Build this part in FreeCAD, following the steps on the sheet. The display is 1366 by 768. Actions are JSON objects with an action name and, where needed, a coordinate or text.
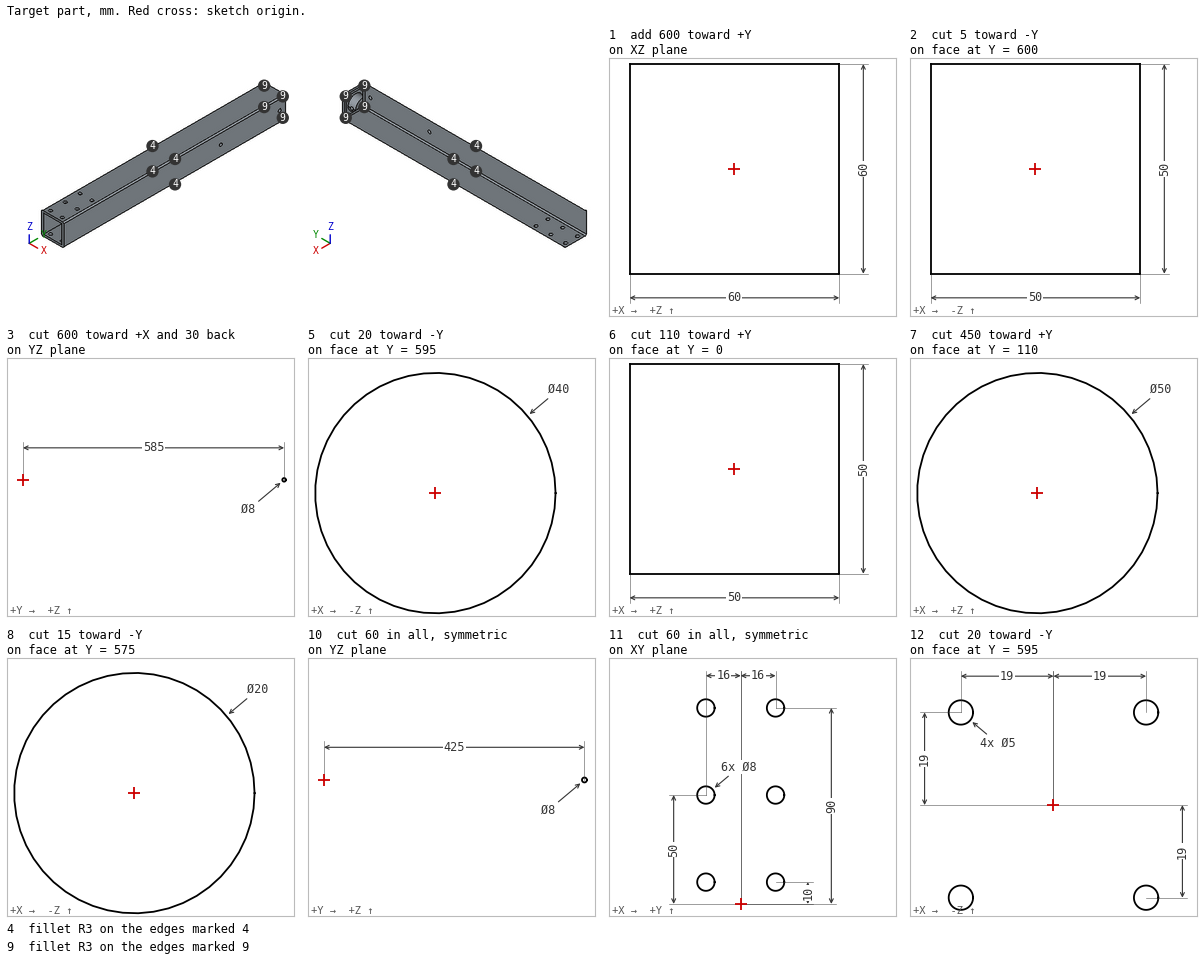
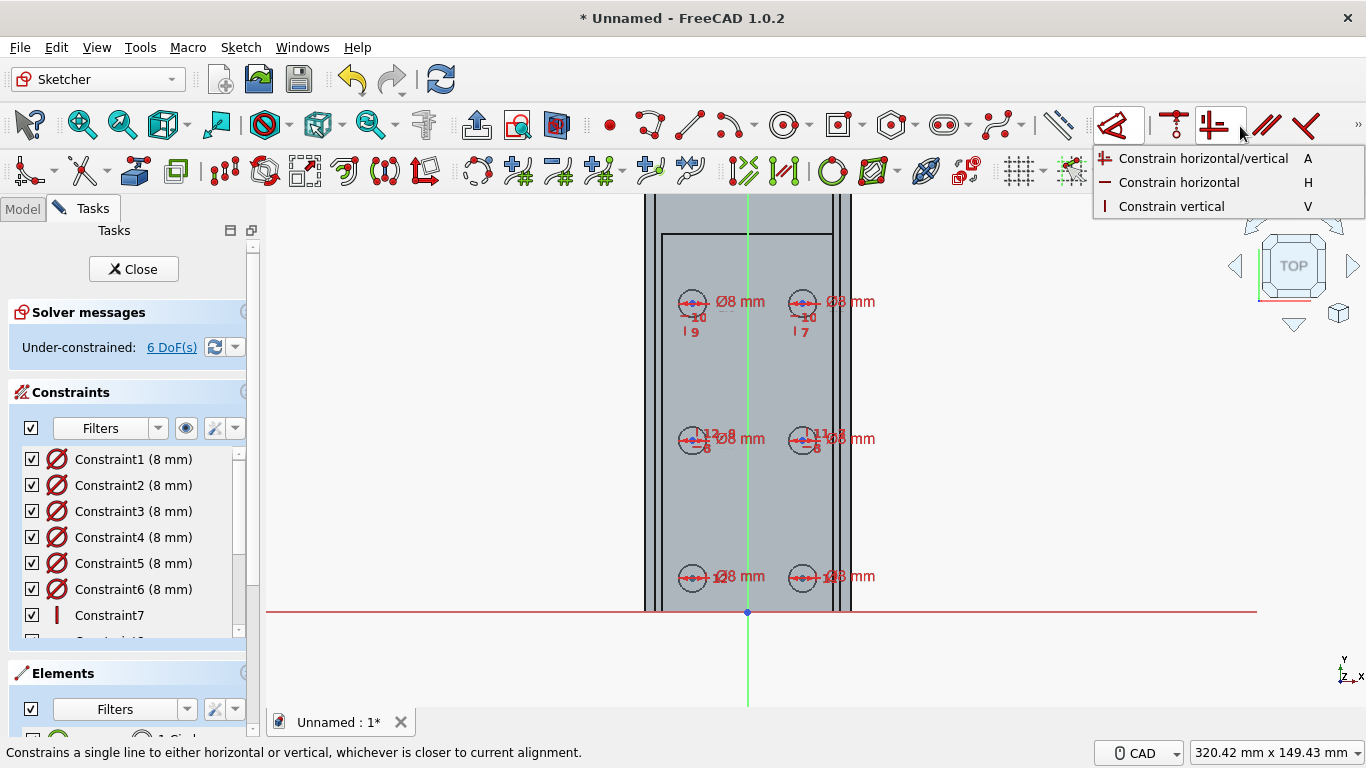
{"action": "left_click", "coordinate": [1229, 182]}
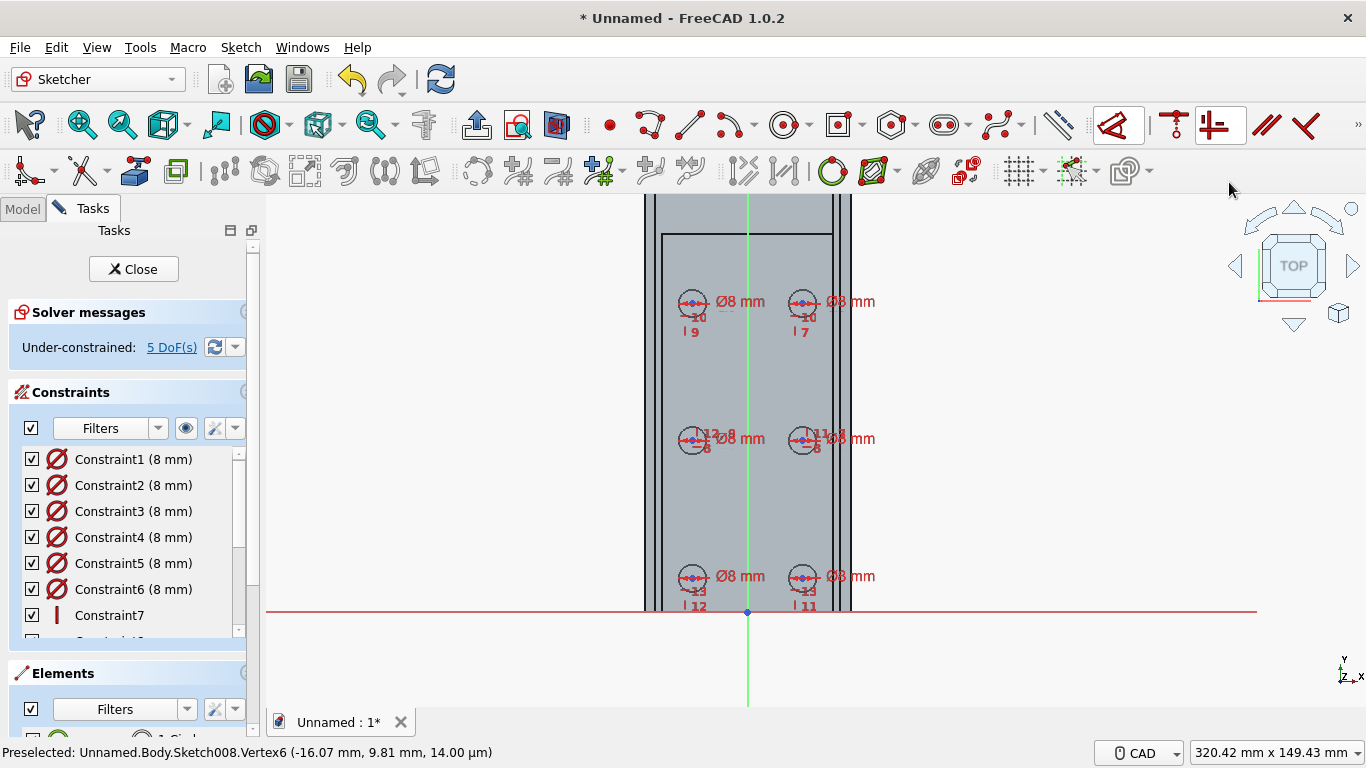
{"action": "left_click", "coordinate": [692, 441]}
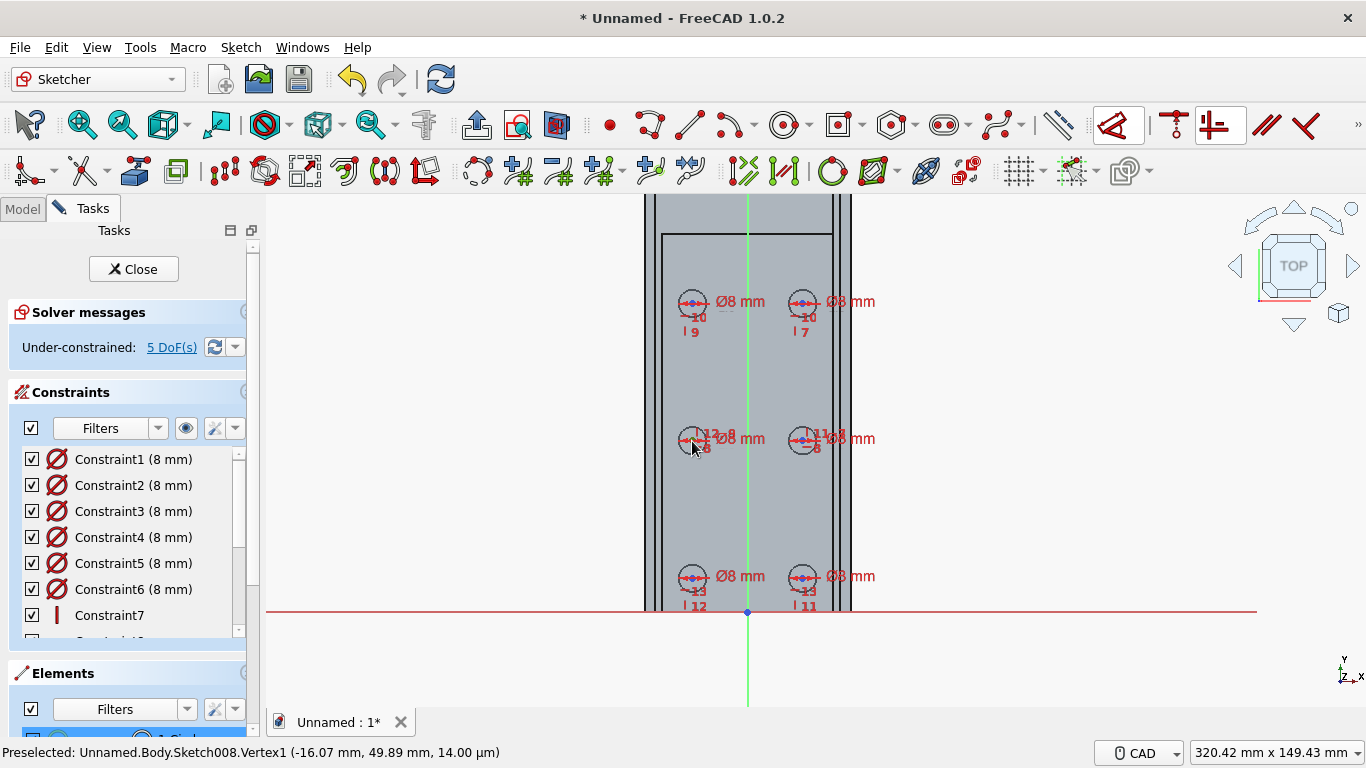
{"action": "key", "text": "l"}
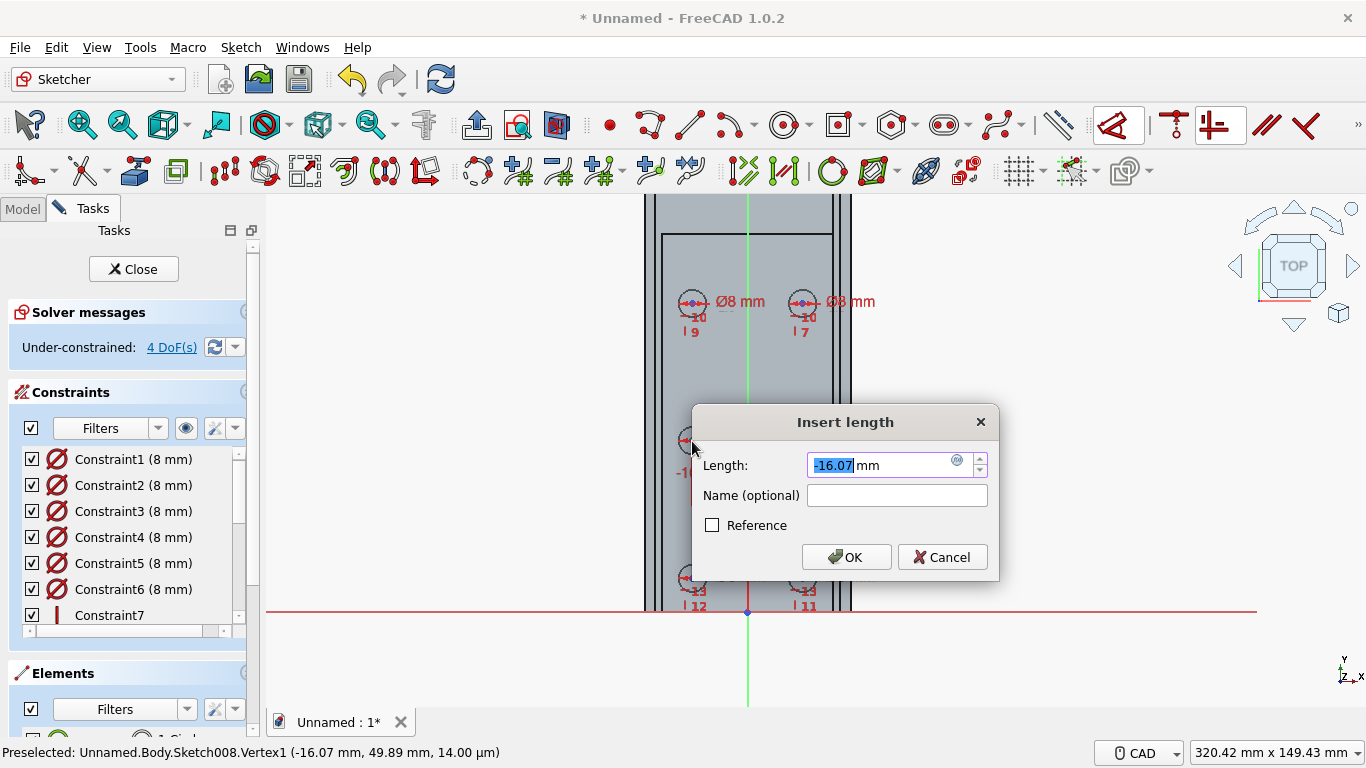
{"action": "type", "text": "-16"}
{"action": "key", "text": "Return"}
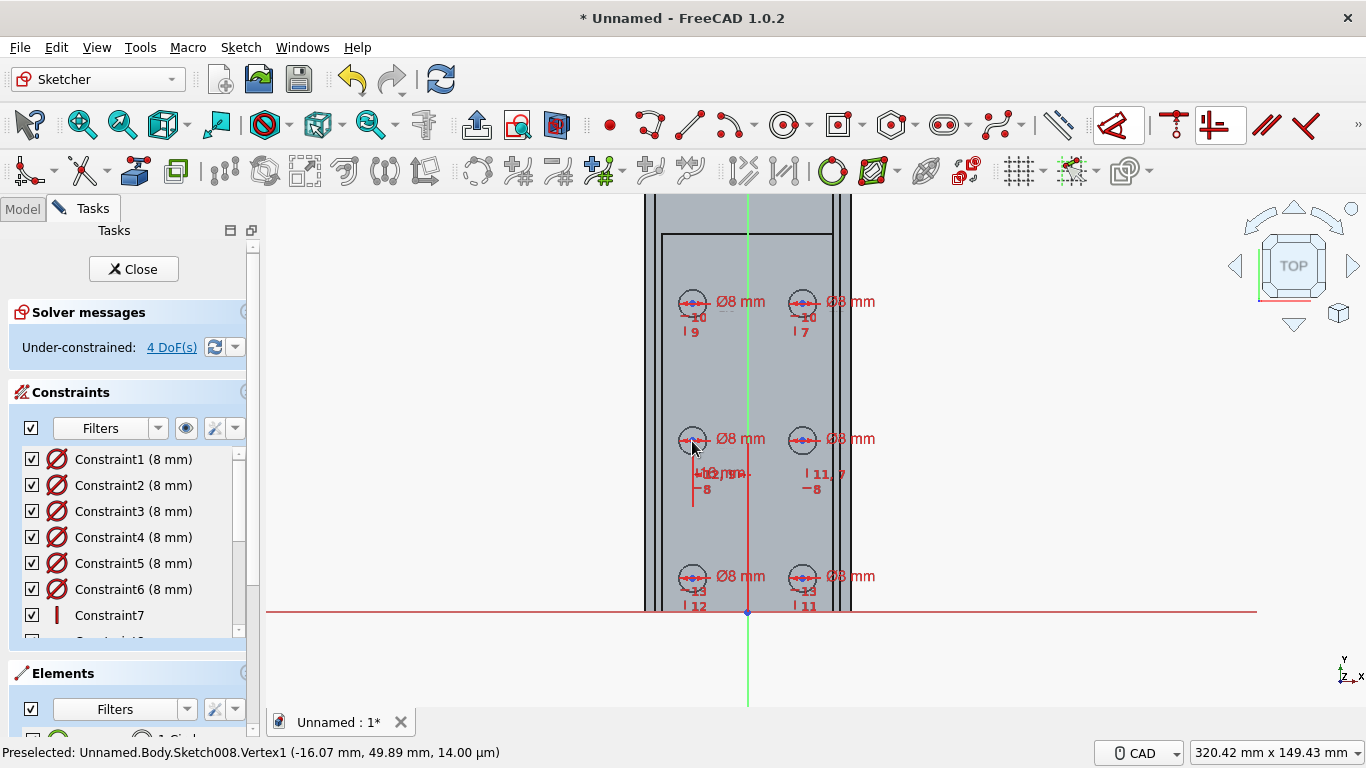
{"action": "left_click", "coordinate": [693, 441]}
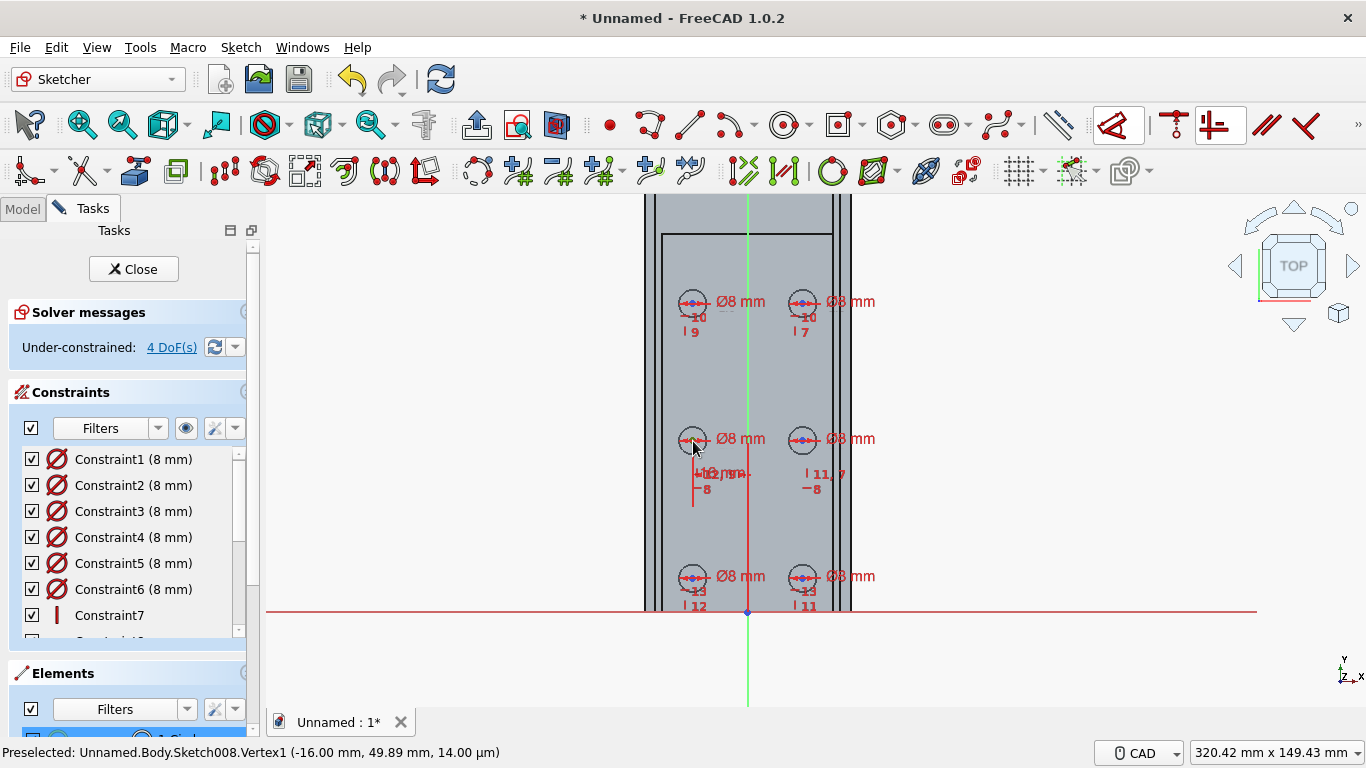
{"action": "key", "text": "i"}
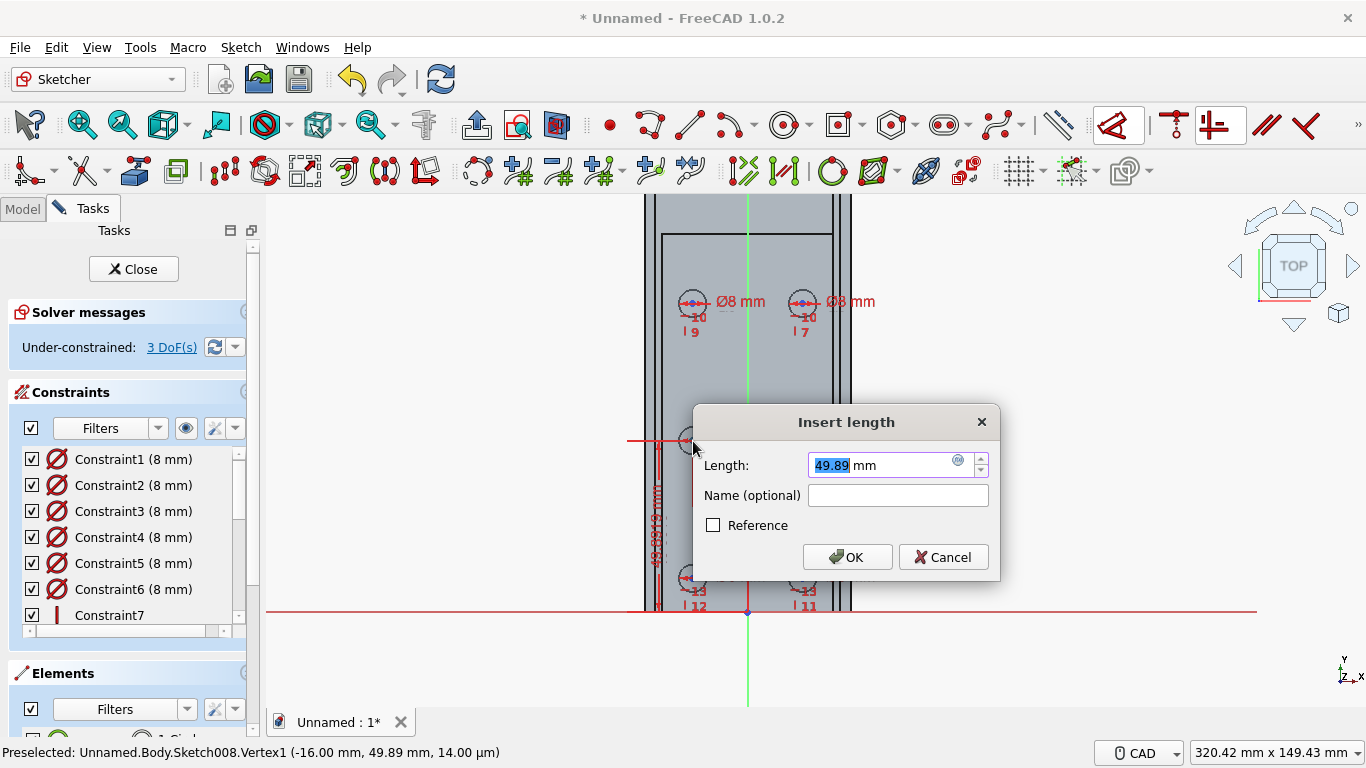
{"action": "type", "text": "50"}
{"action": "key", "text": "Return"}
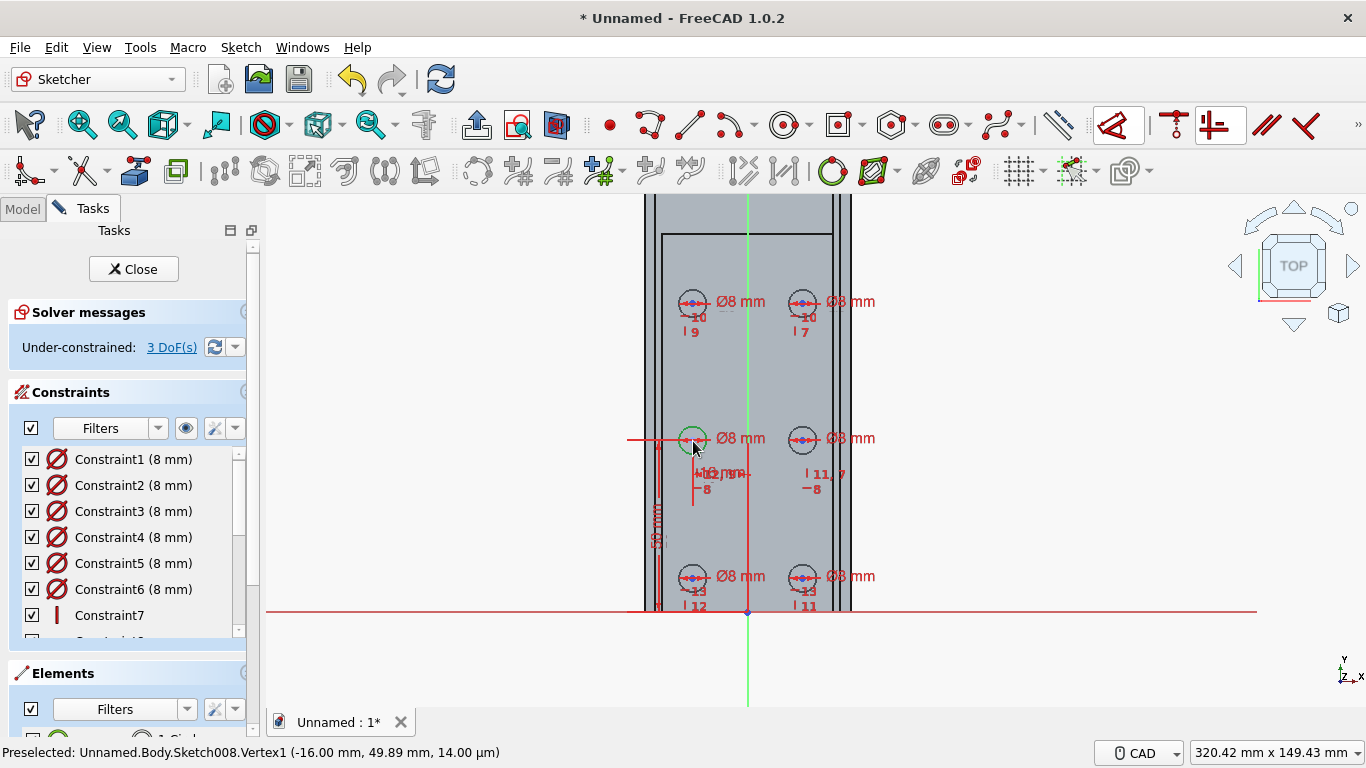
{"action": "left_click", "coordinate": [803, 304]}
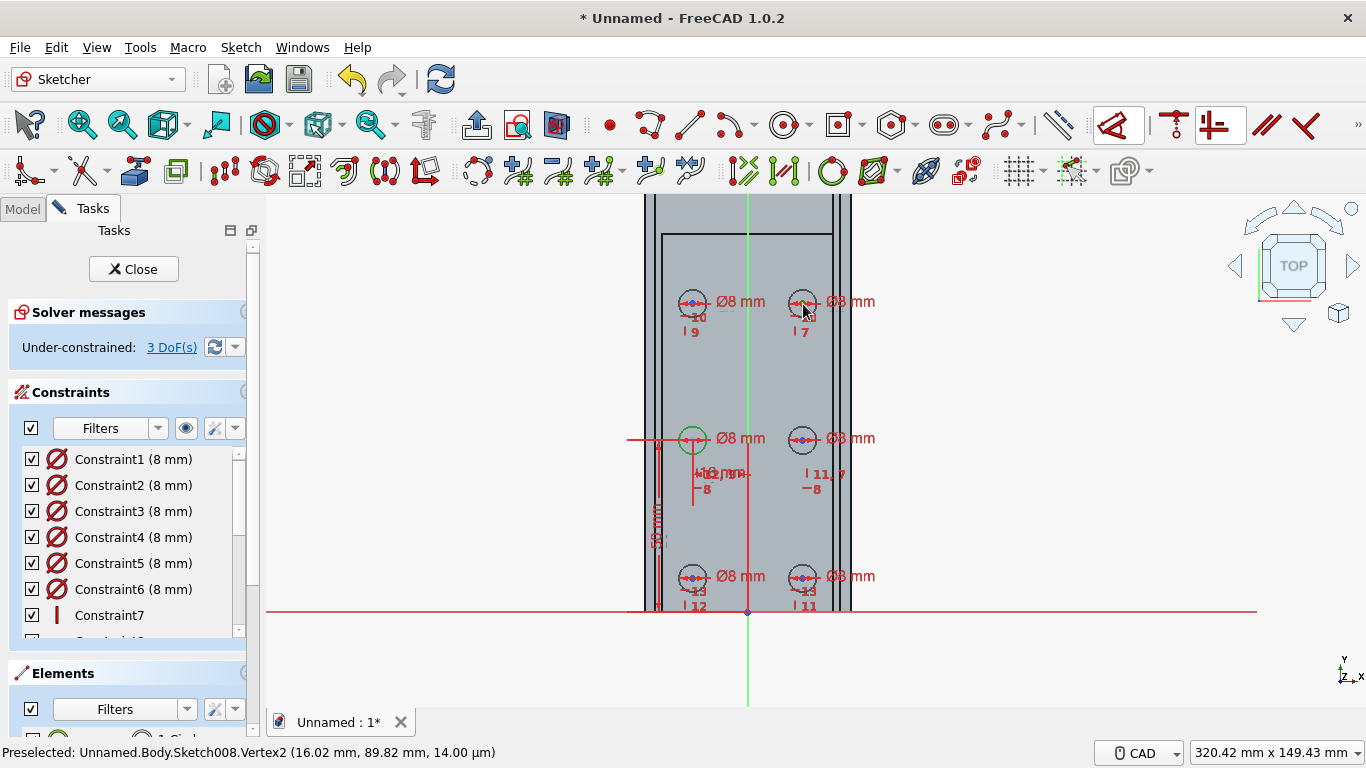
{"action": "left_click", "coordinate": [1138, 126]}